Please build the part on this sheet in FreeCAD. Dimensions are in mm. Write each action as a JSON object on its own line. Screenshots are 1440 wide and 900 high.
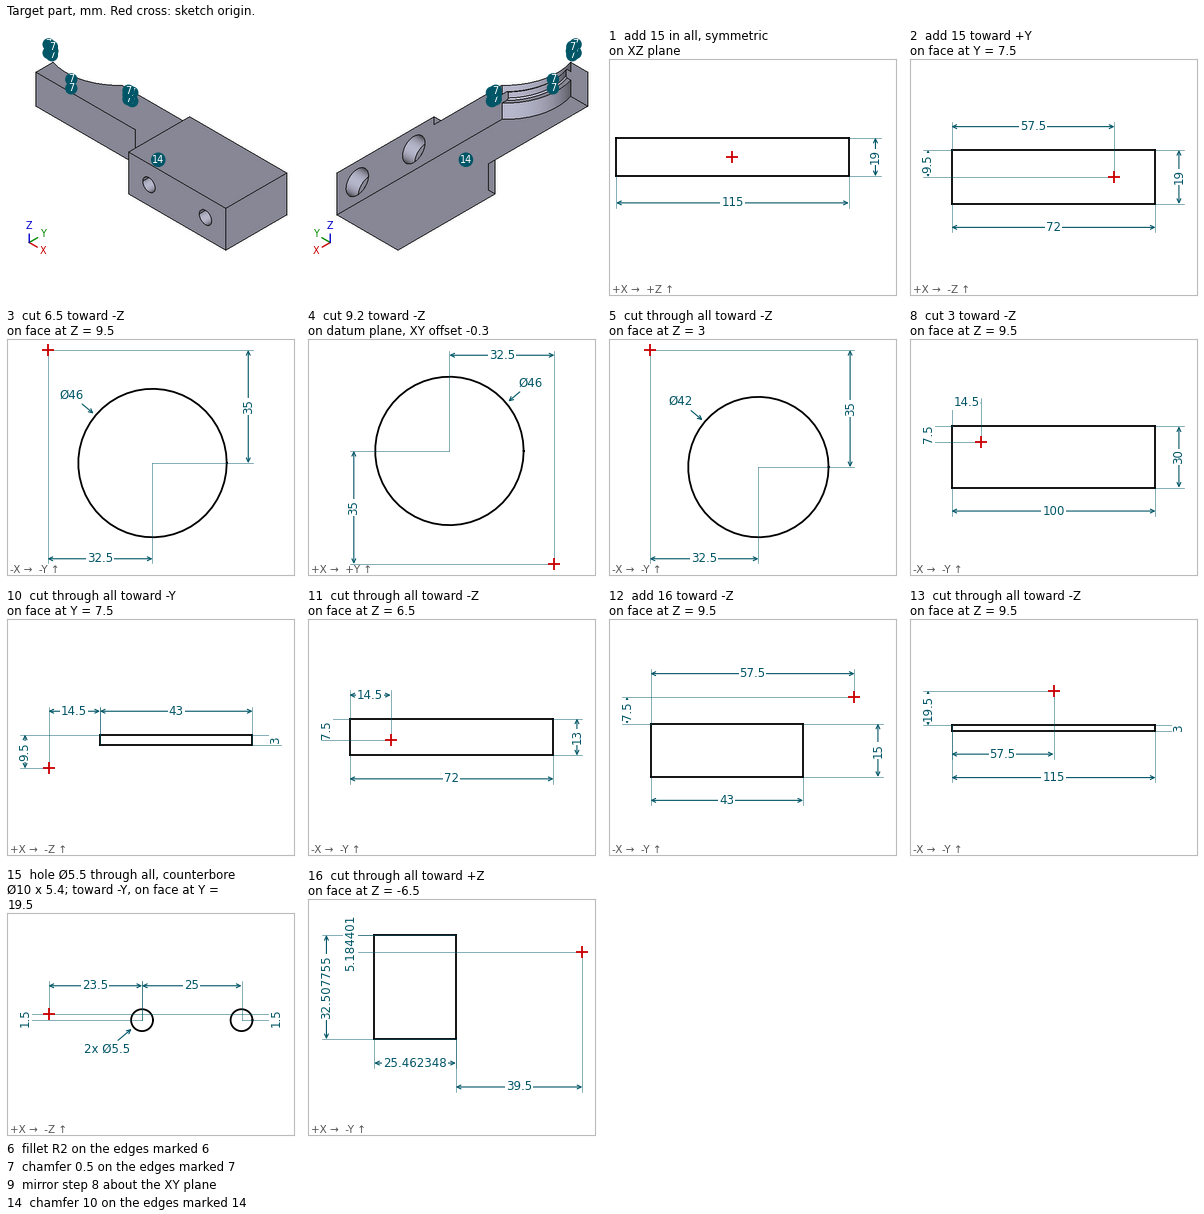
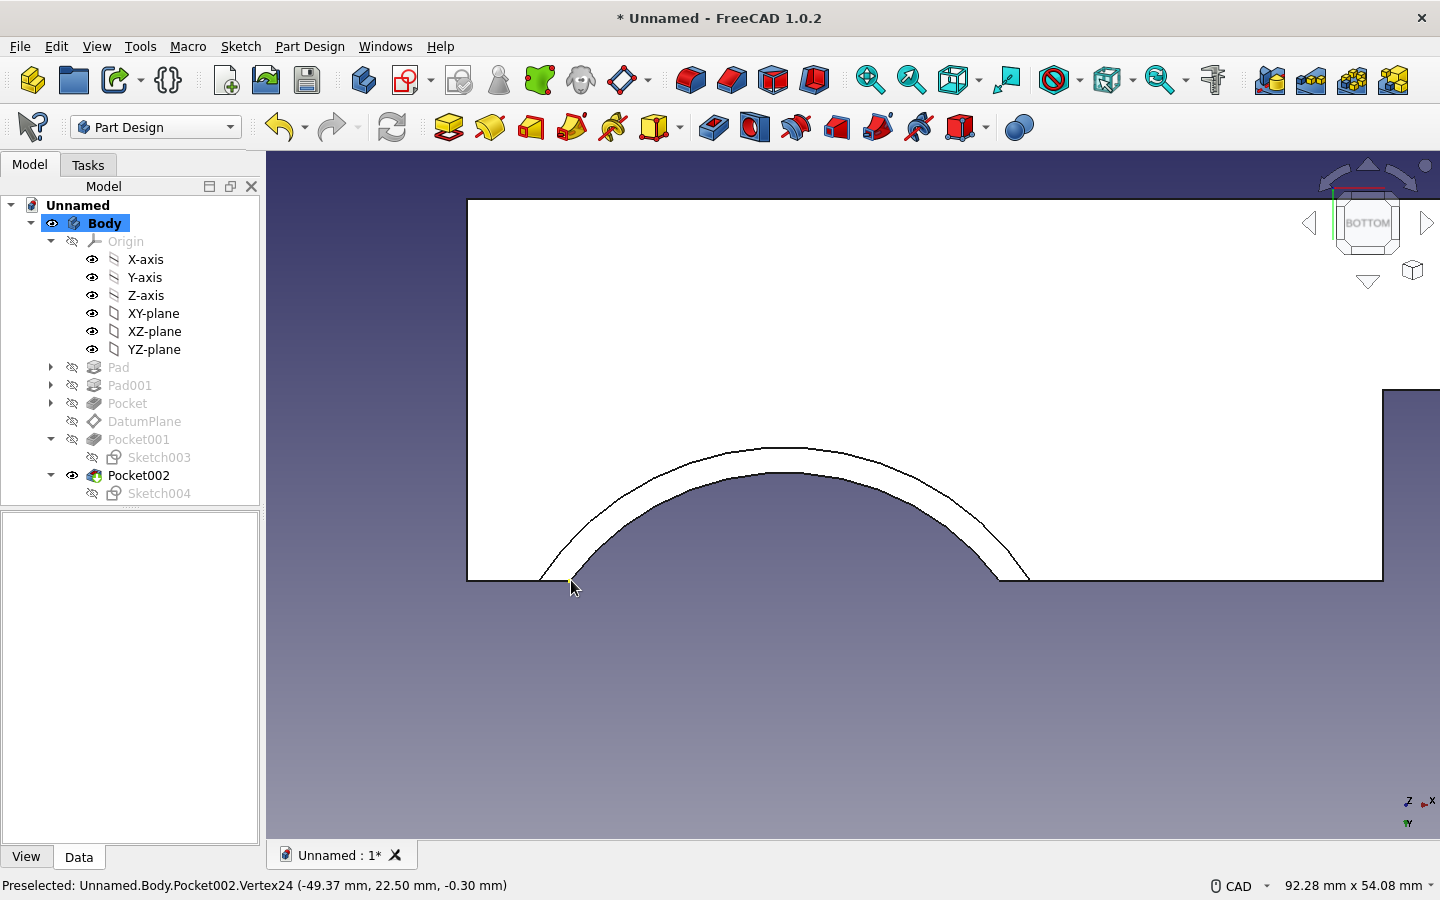
{"action": "left_click", "coordinate": [871, 80]}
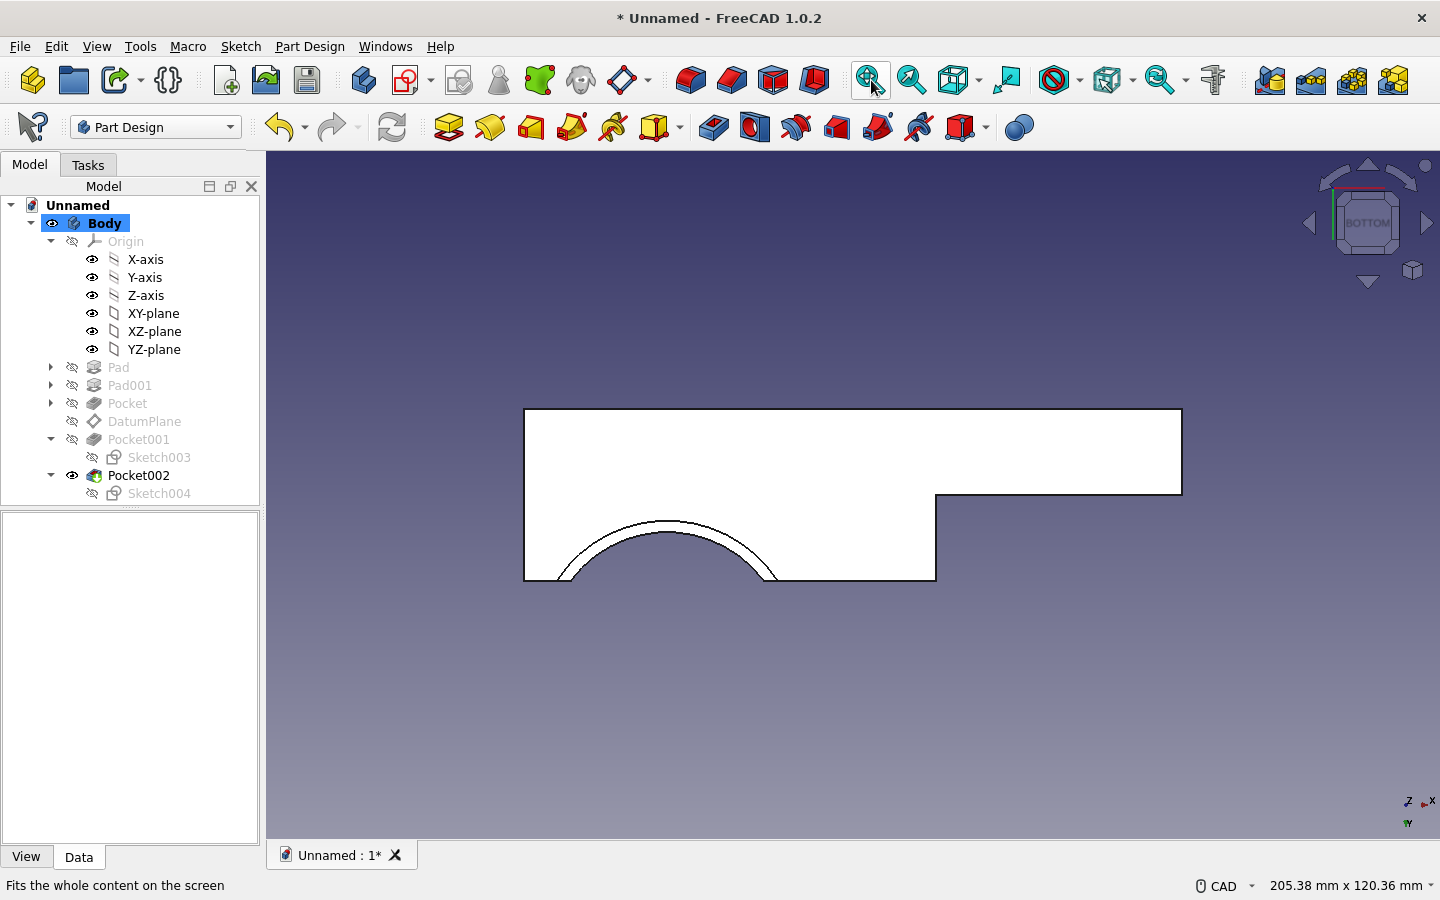
{"action": "key", "text": "4"}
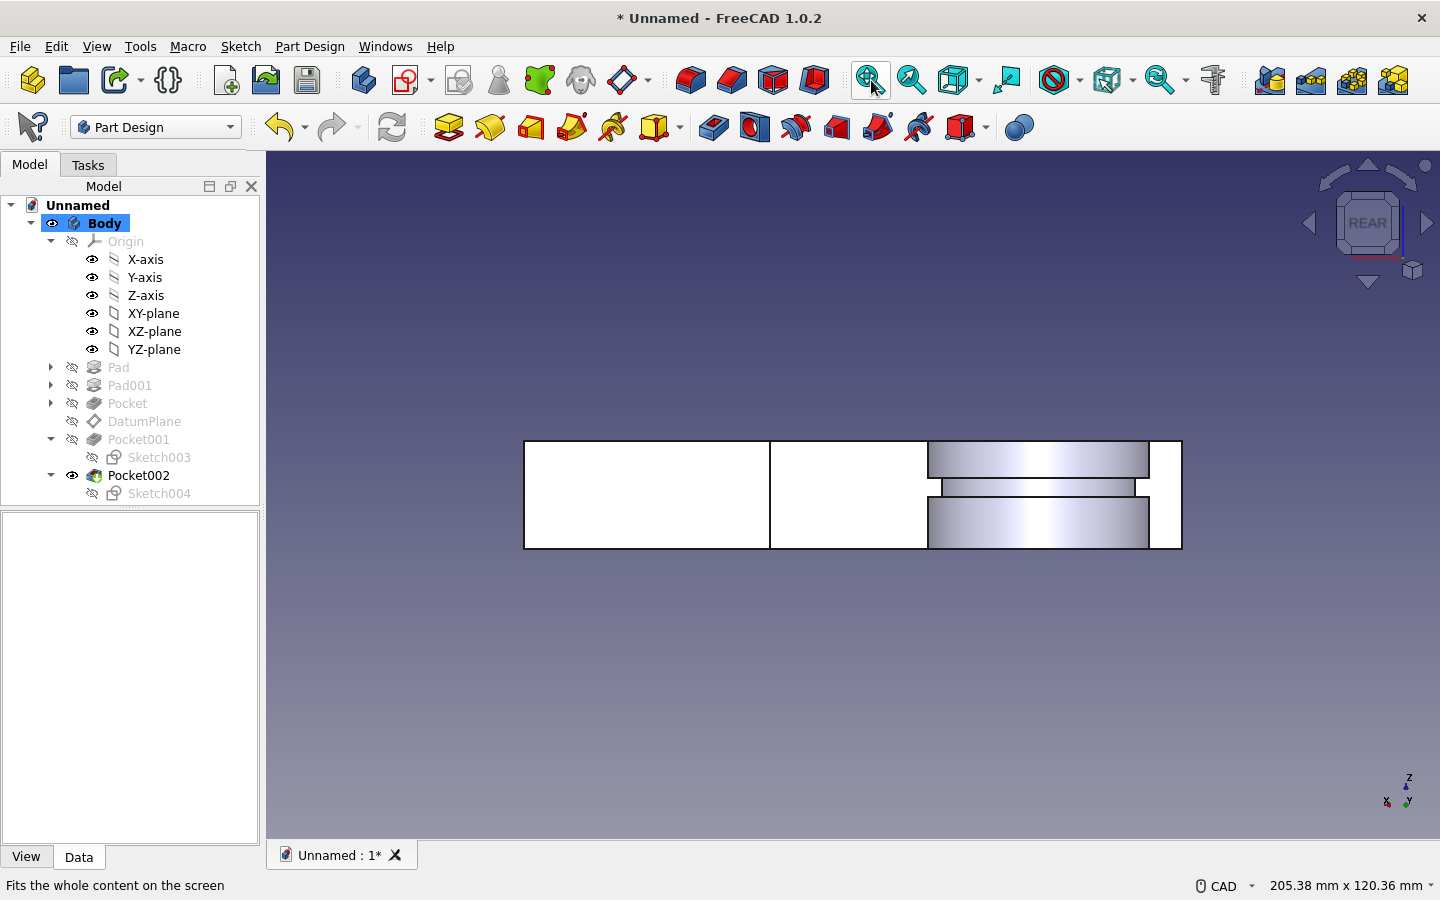
{"action": "left_click", "coordinate": [1135, 486]}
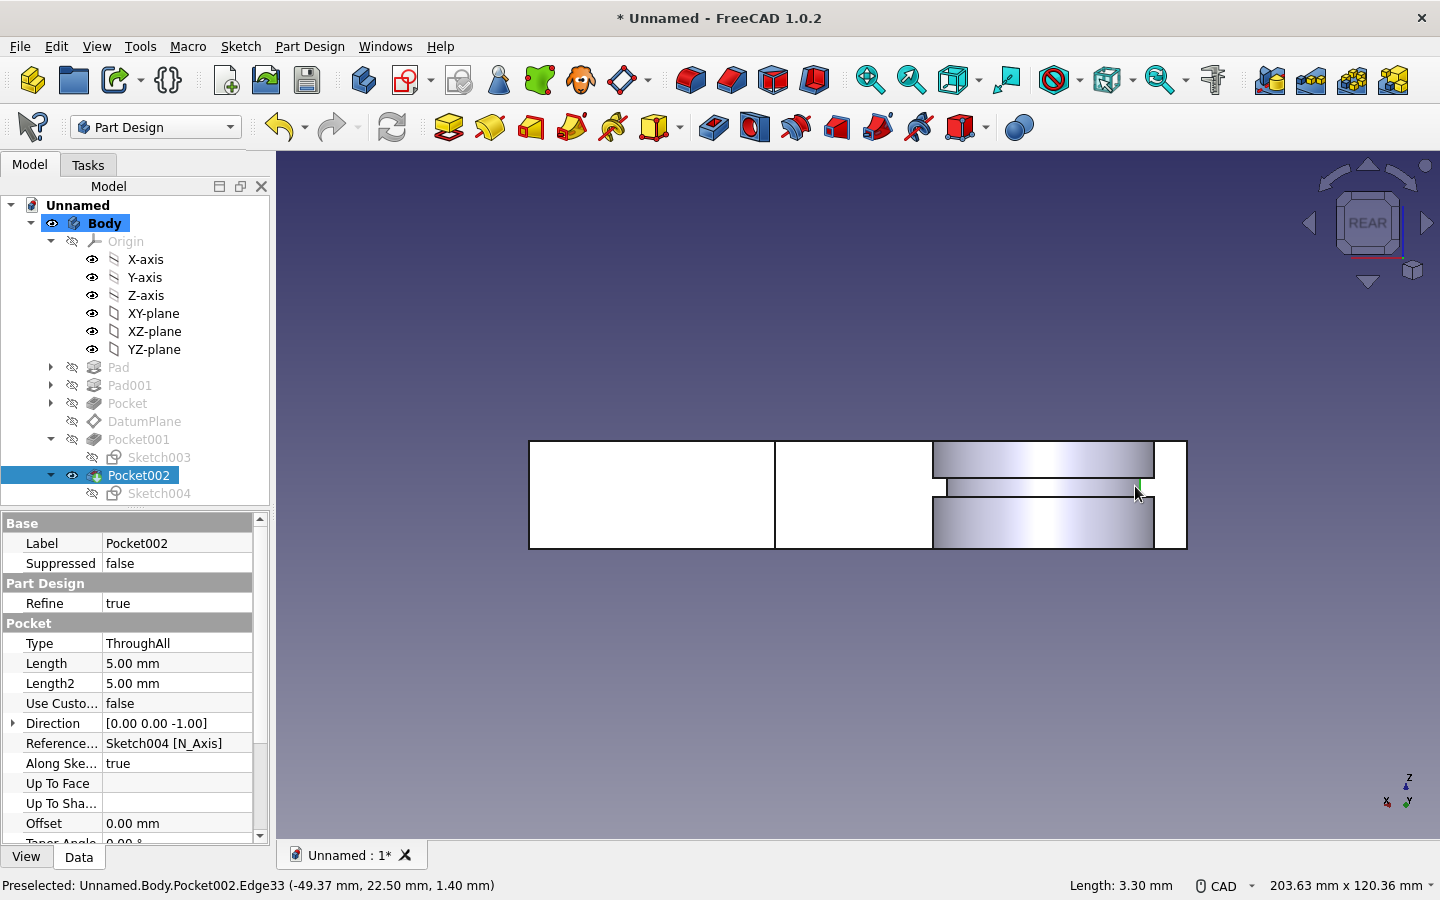
{"action": "left_click", "coordinate": [947, 486], "text": "ctrl"}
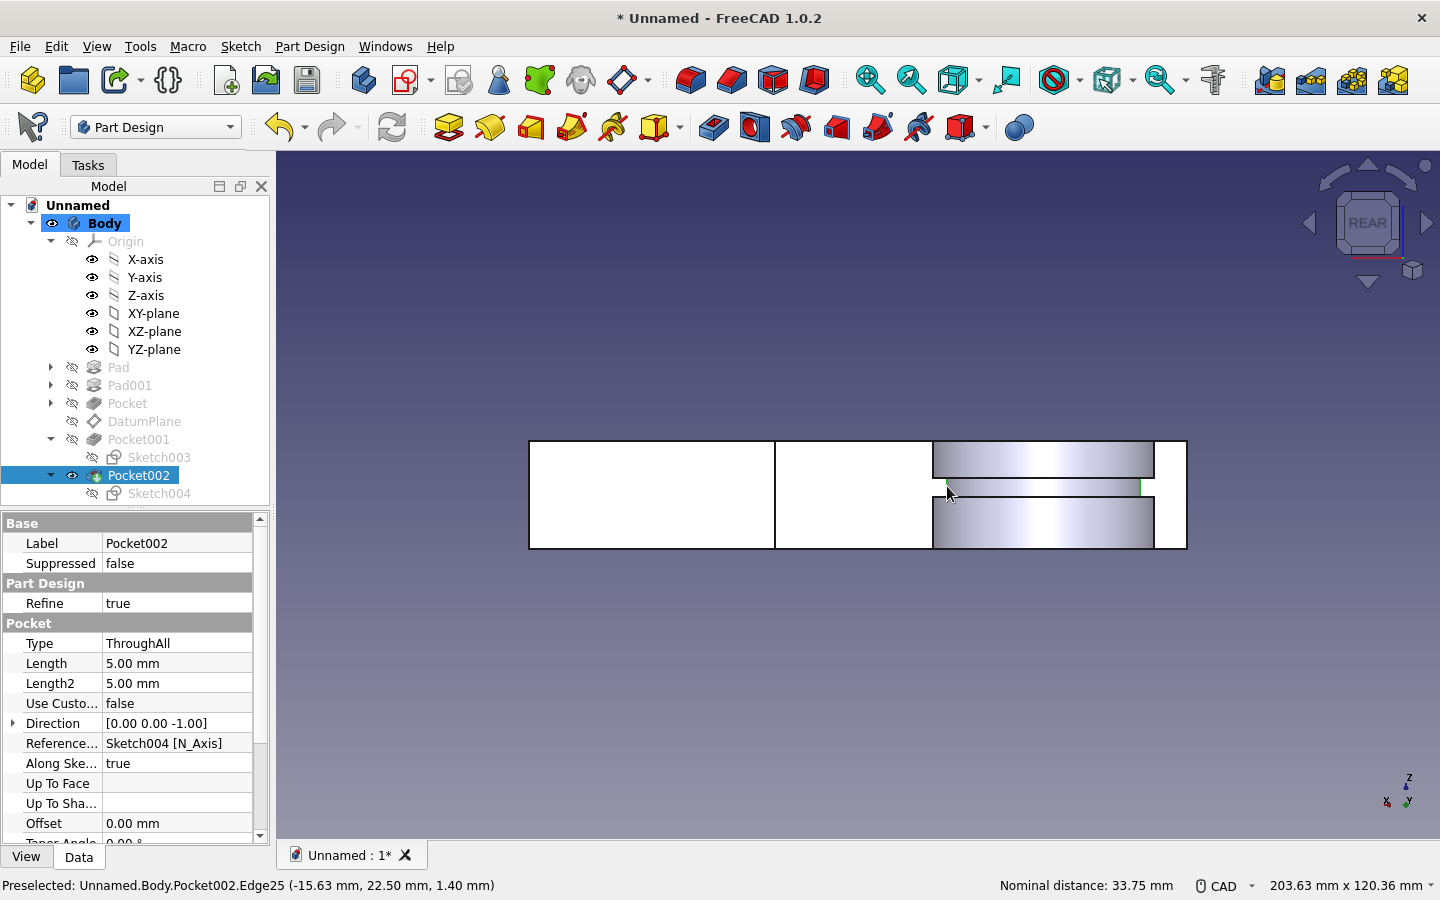
{"action": "left_click", "coordinate": [691, 80]}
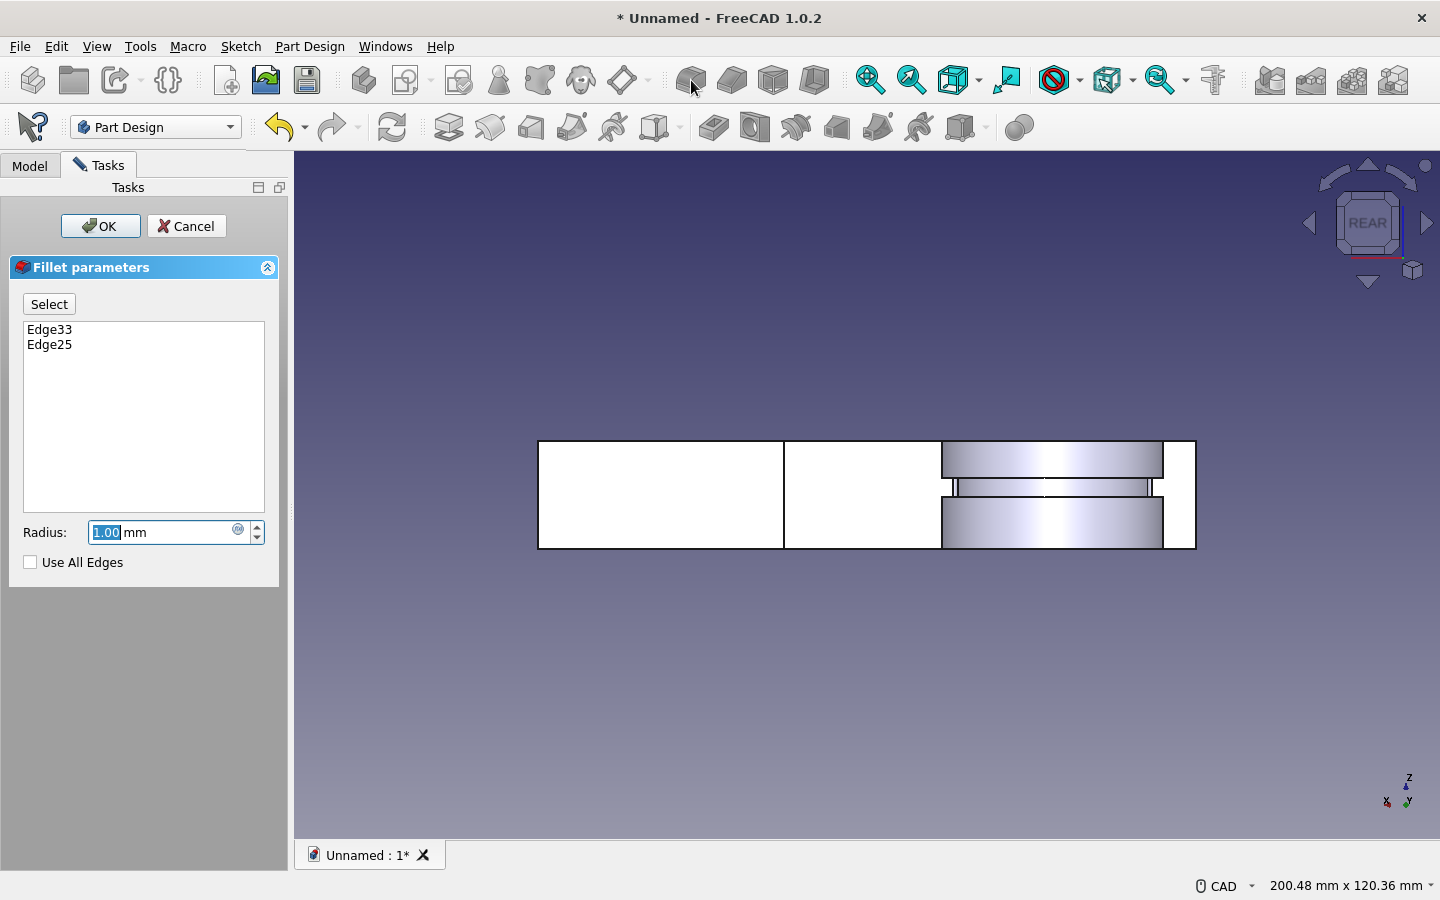
{"action": "type", "text": "2"}
{"action": "key", "text": "Tab"}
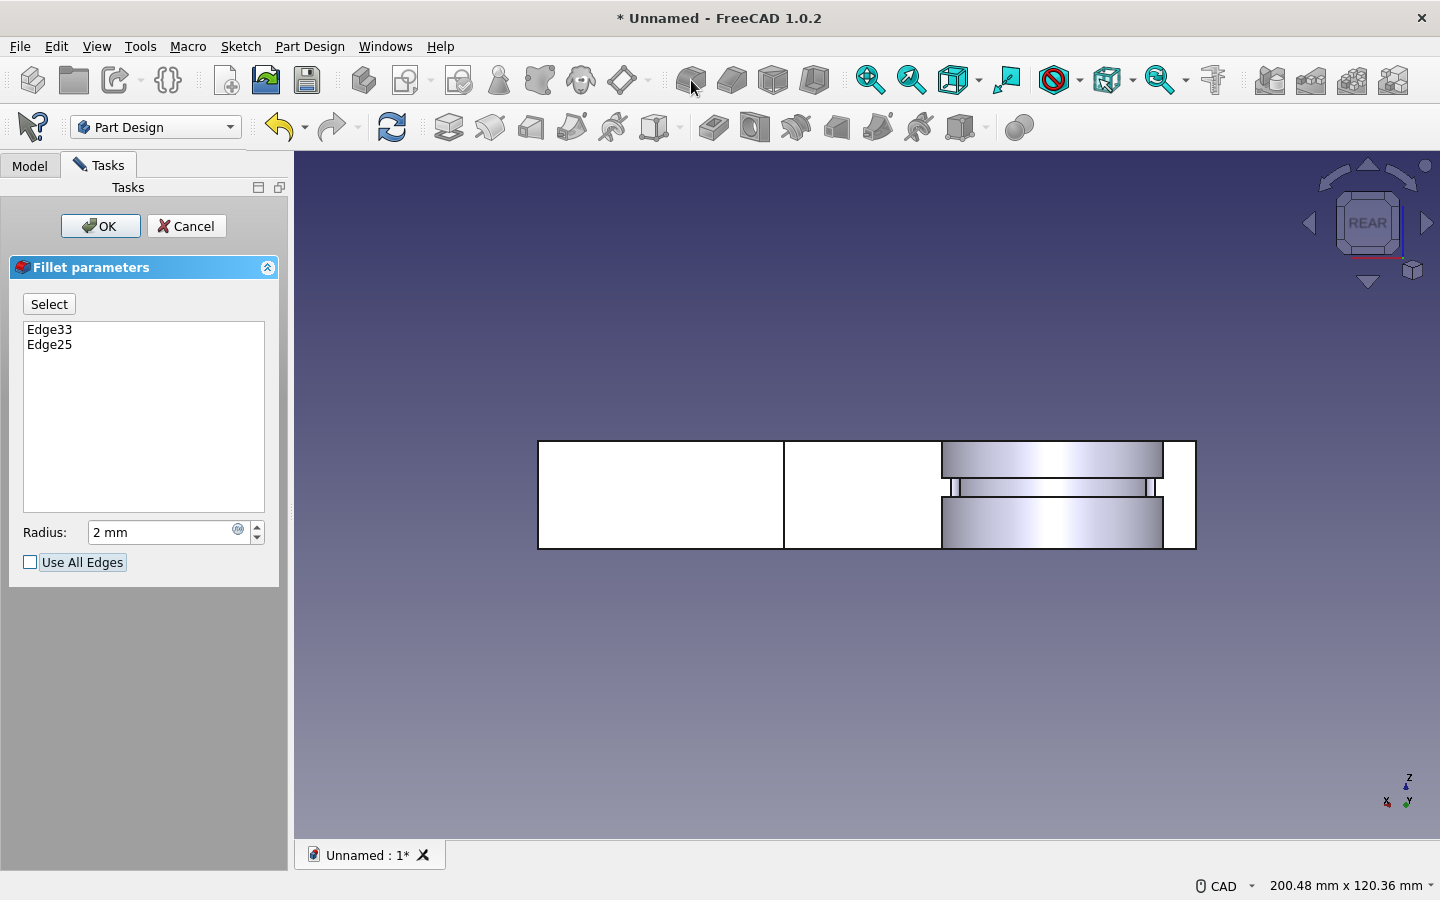
{"action": "left_click", "coordinate": [101, 226]}